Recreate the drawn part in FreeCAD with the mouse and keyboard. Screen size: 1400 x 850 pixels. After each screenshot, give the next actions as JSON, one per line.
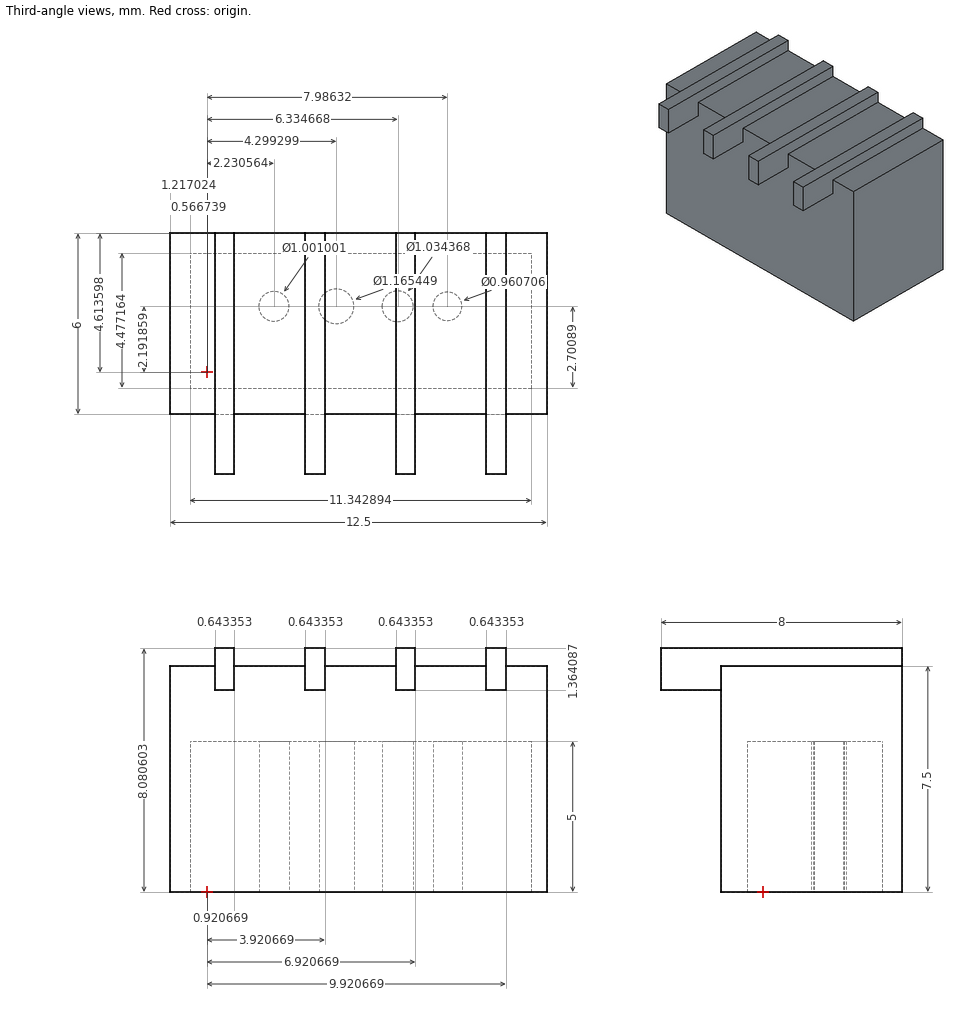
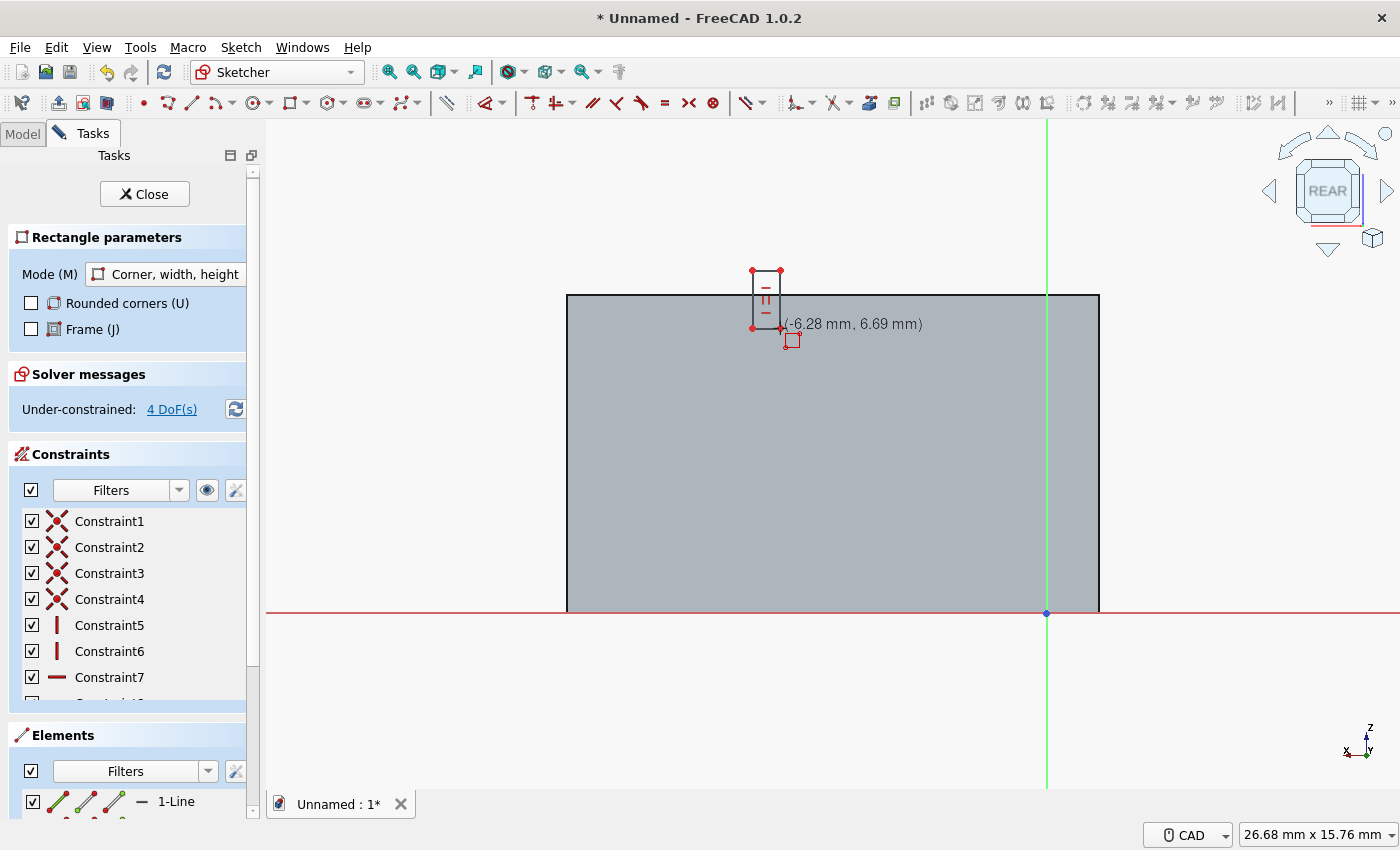
{"action": "left_click", "coordinate": [625, 270]}
{"action": "left_click", "coordinate": [653, 328]}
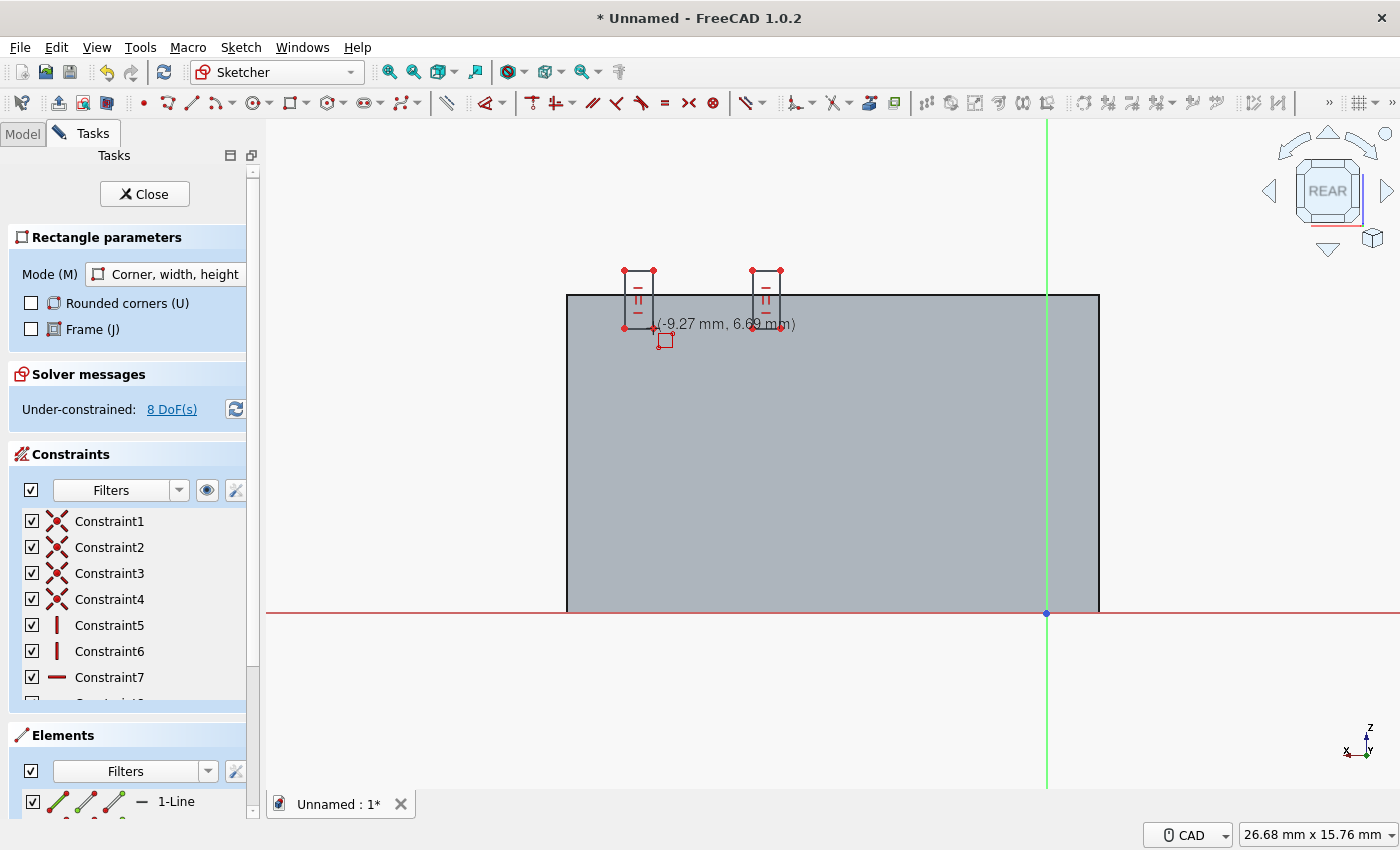
{"action": "left_click", "coordinate": [880, 270]}
{"action": "left_click", "coordinate": [908, 328]}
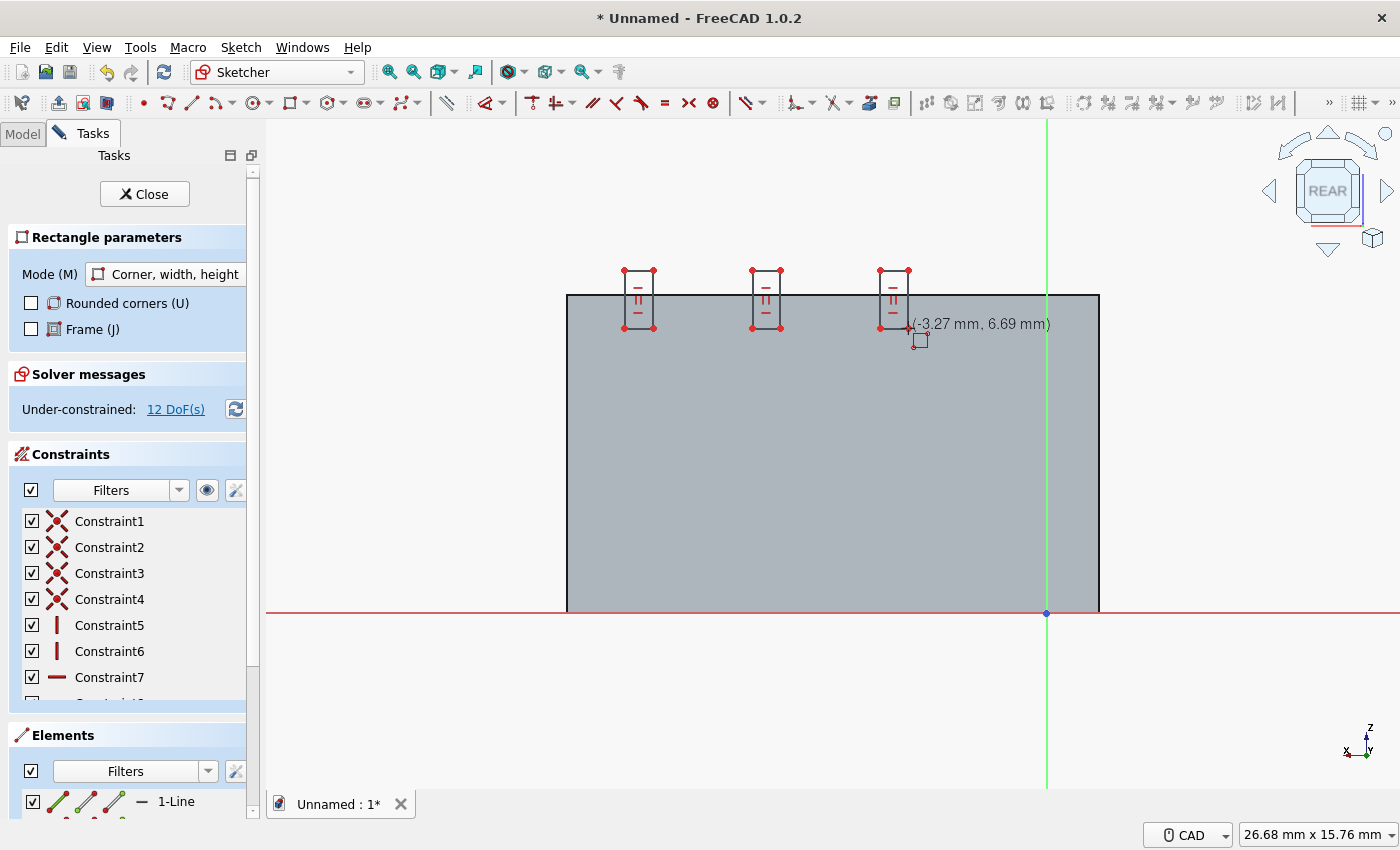
{"action": "left_click", "coordinate": [1008, 270]}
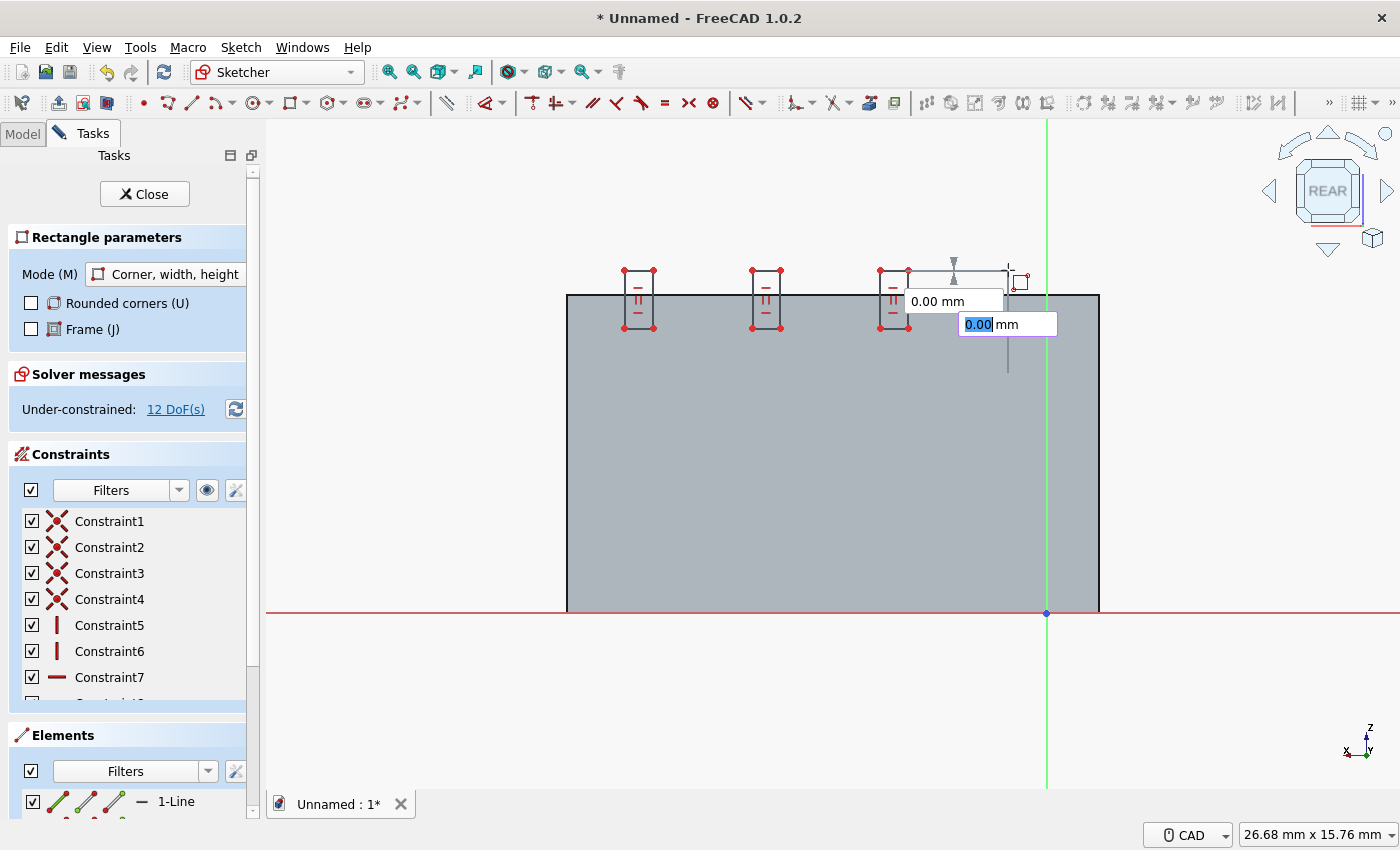
{"action": "scroll", "coordinate": [1035, 328], "scroll_direction": "up", "scroll_amount": 2}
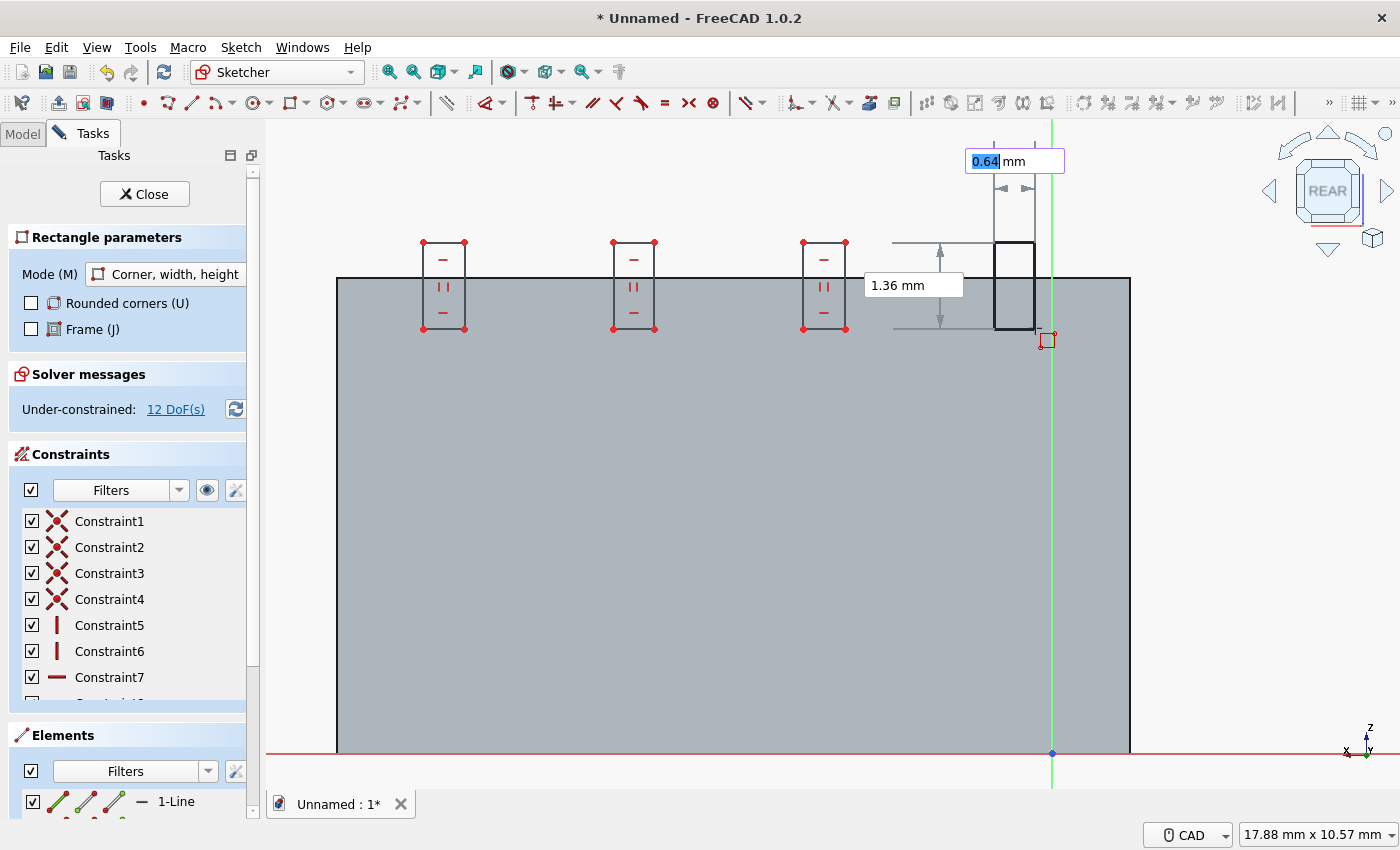
{"action": "left_click", "coordinate": [1035, 328]}
{"action": "key", "text": "Escape"}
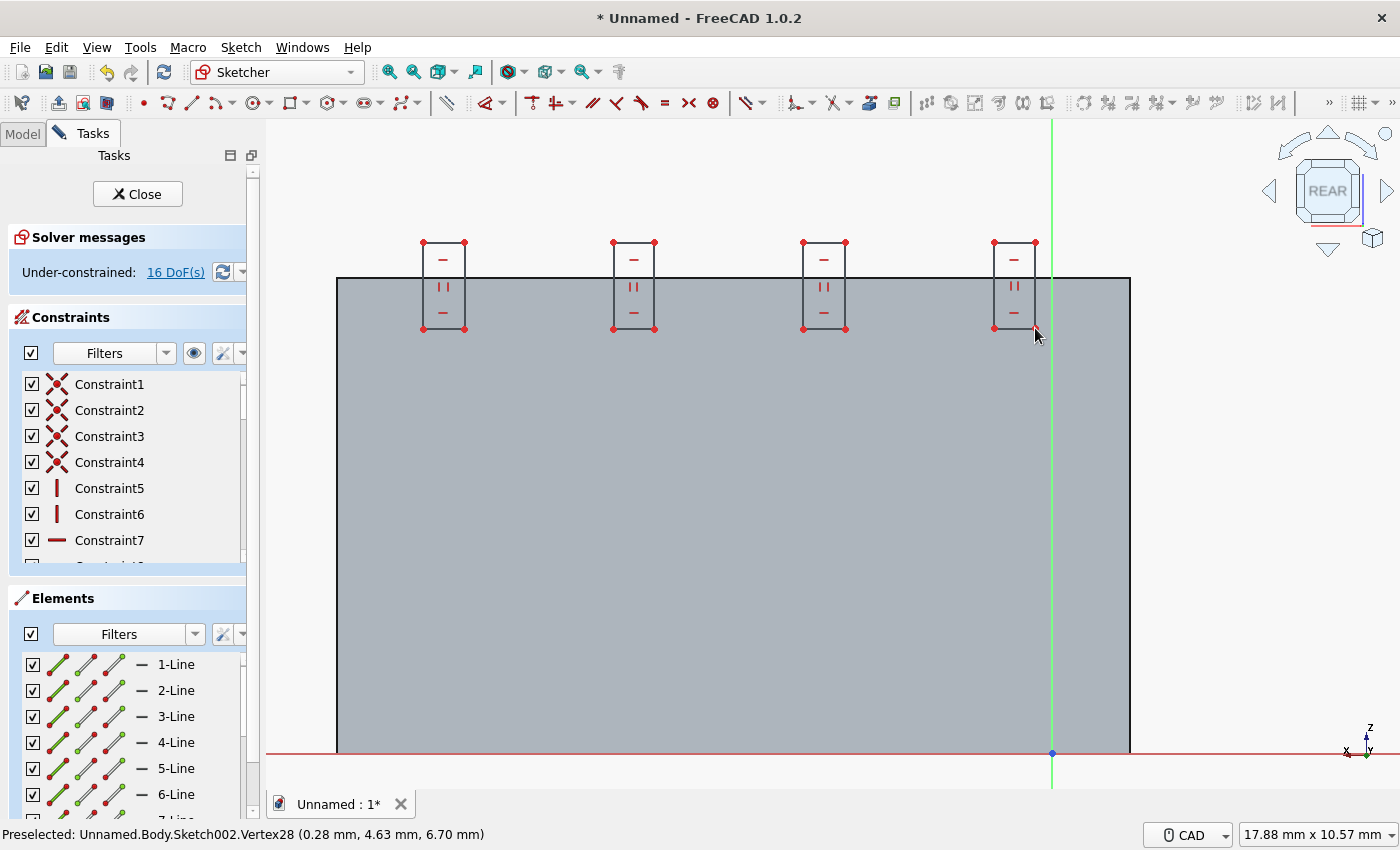
{"action": "left_click", "coordinate": [486, 104]}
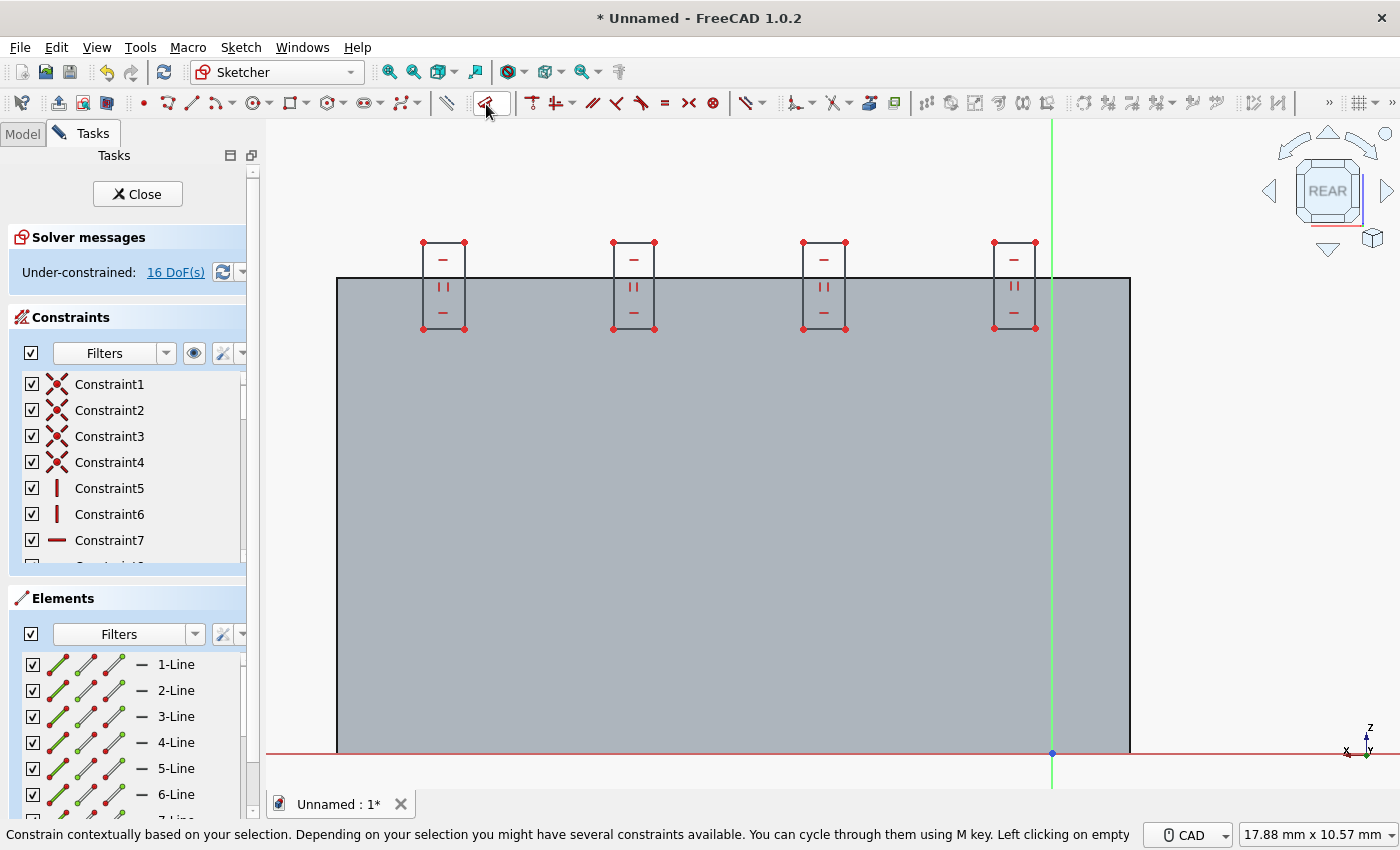
{"action": "left_click", "coordinate": [614, 269]}
{"action": "left_click", "coordinate": [580, 286]}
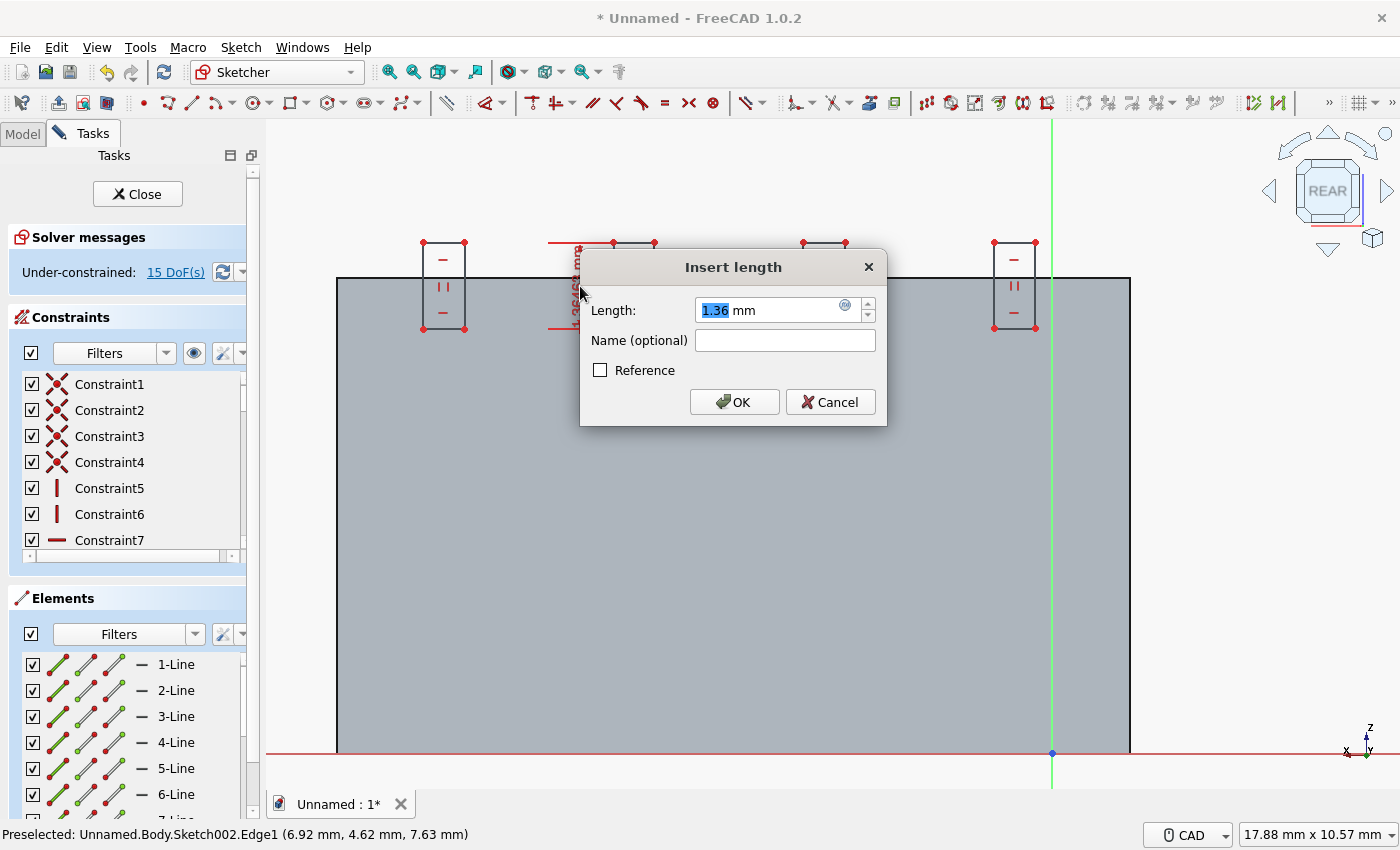
{"action": "type", "text": "1.364087"}
{"action": "key", "text": "Return"}